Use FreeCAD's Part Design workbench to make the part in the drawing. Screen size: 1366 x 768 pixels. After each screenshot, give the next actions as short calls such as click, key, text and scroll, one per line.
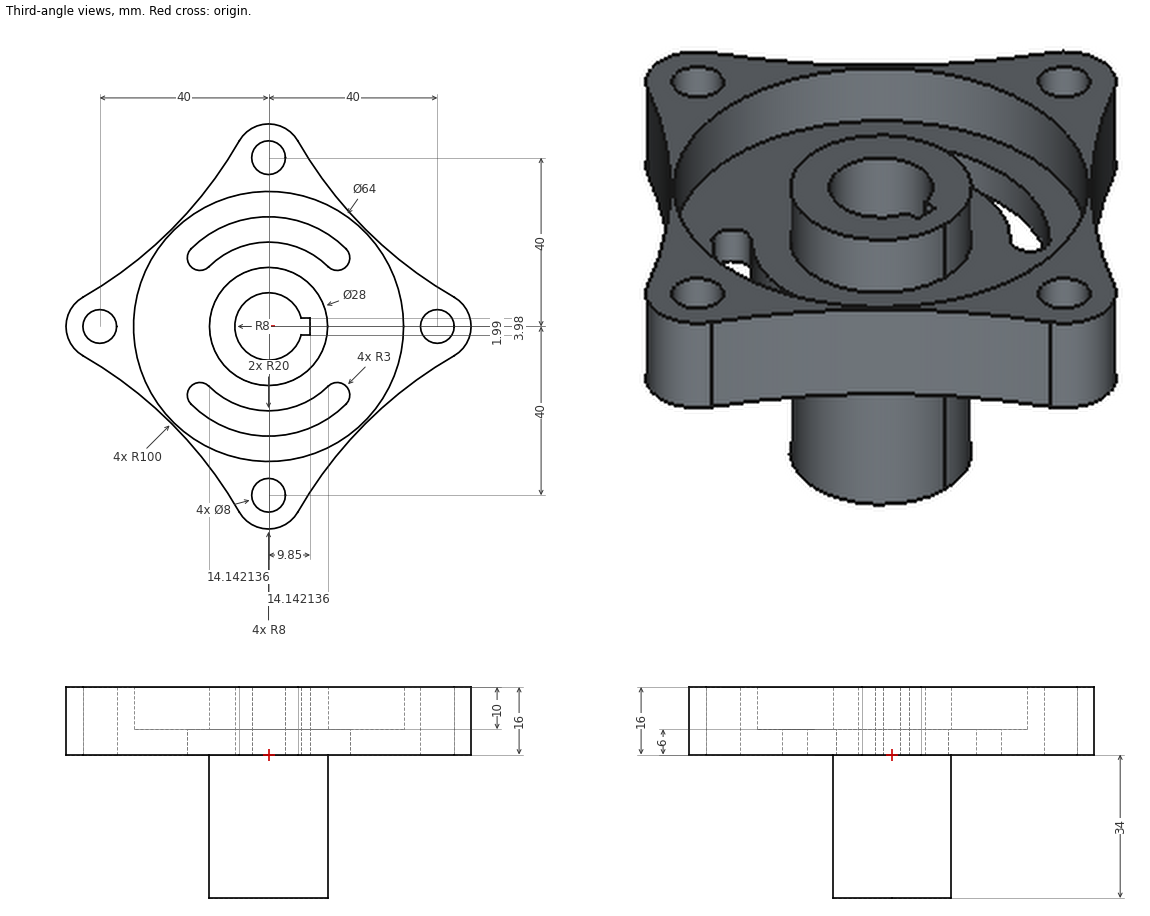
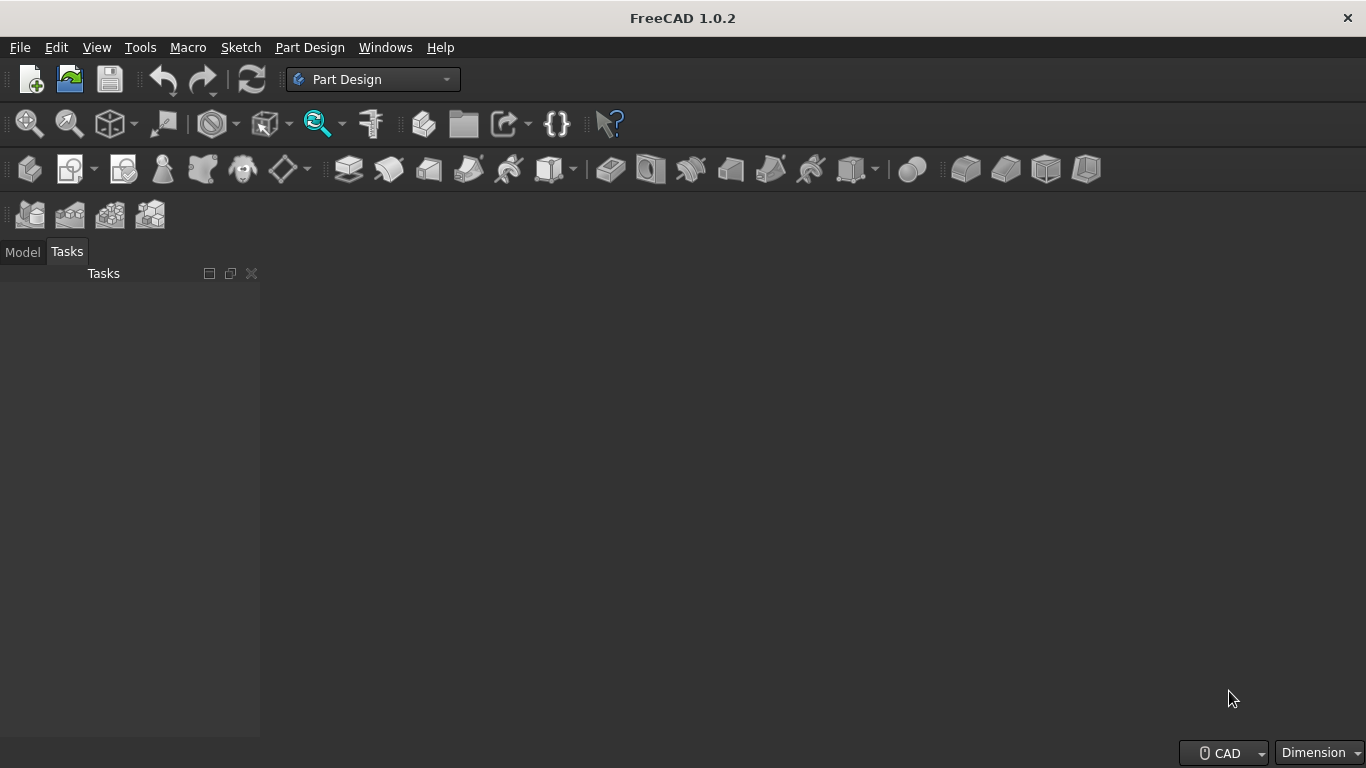
click(30, 80)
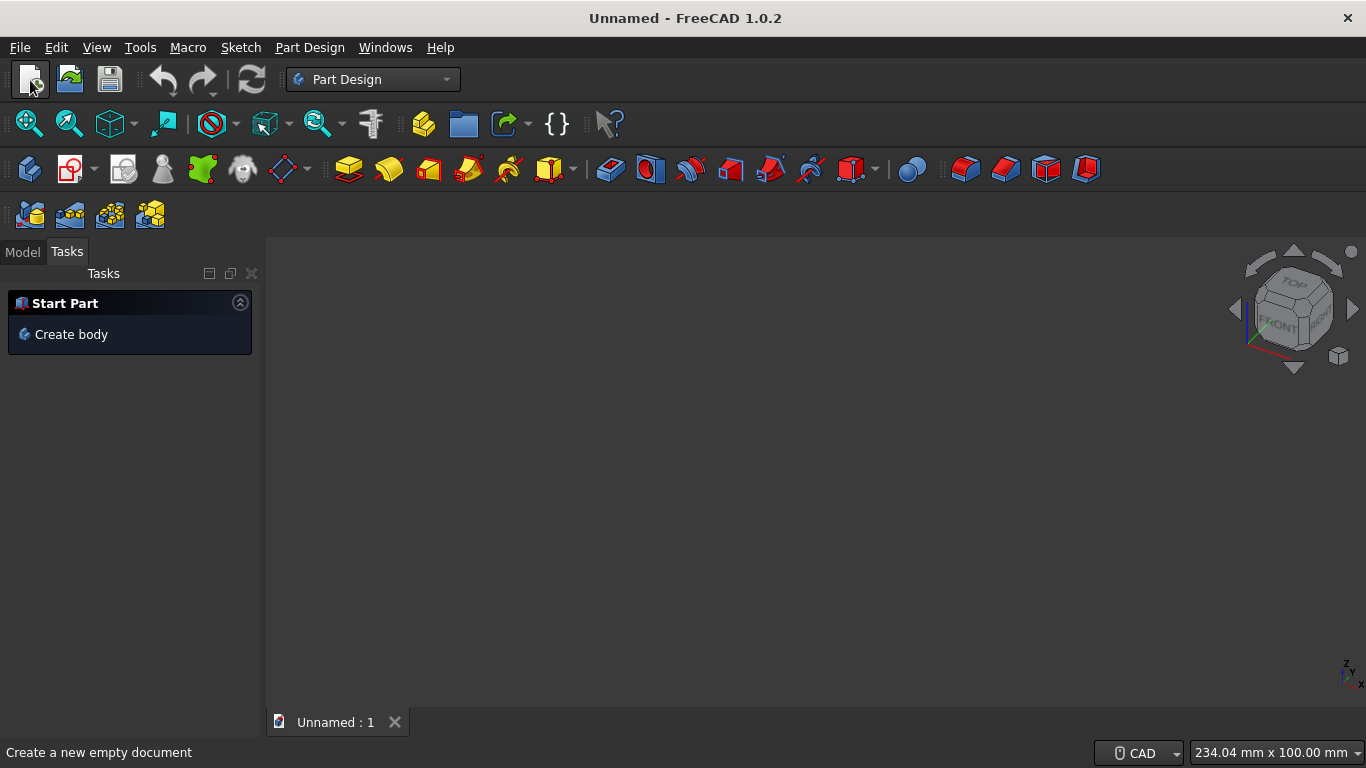
click(70, 170)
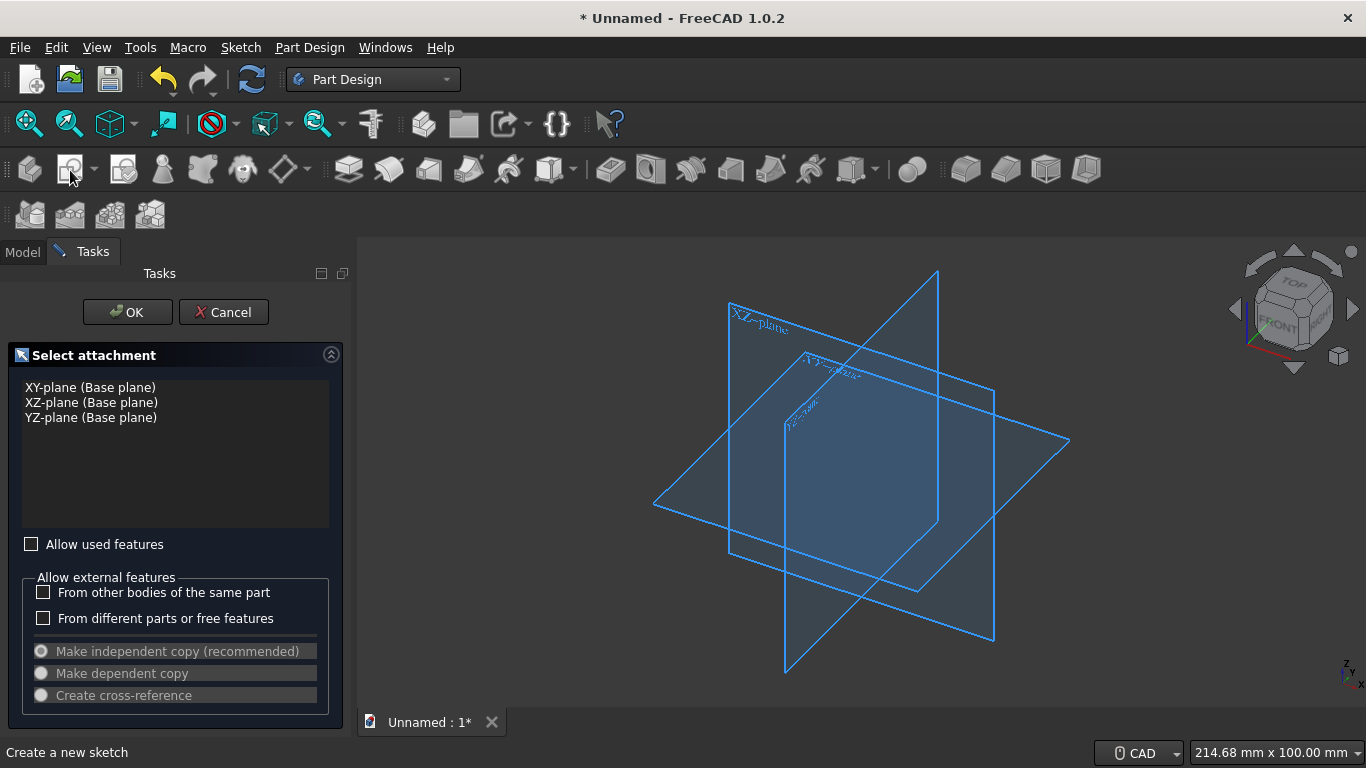
click(82, 388)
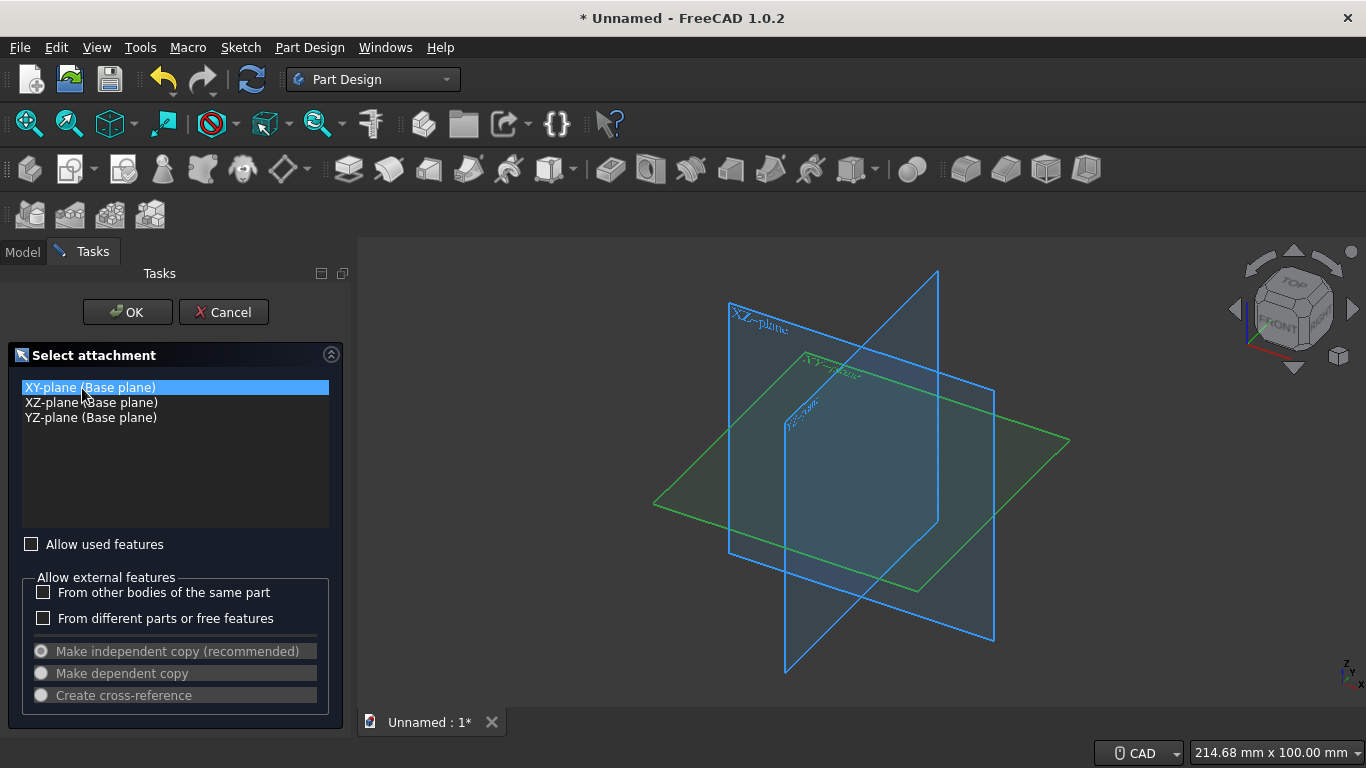
click(128, 312)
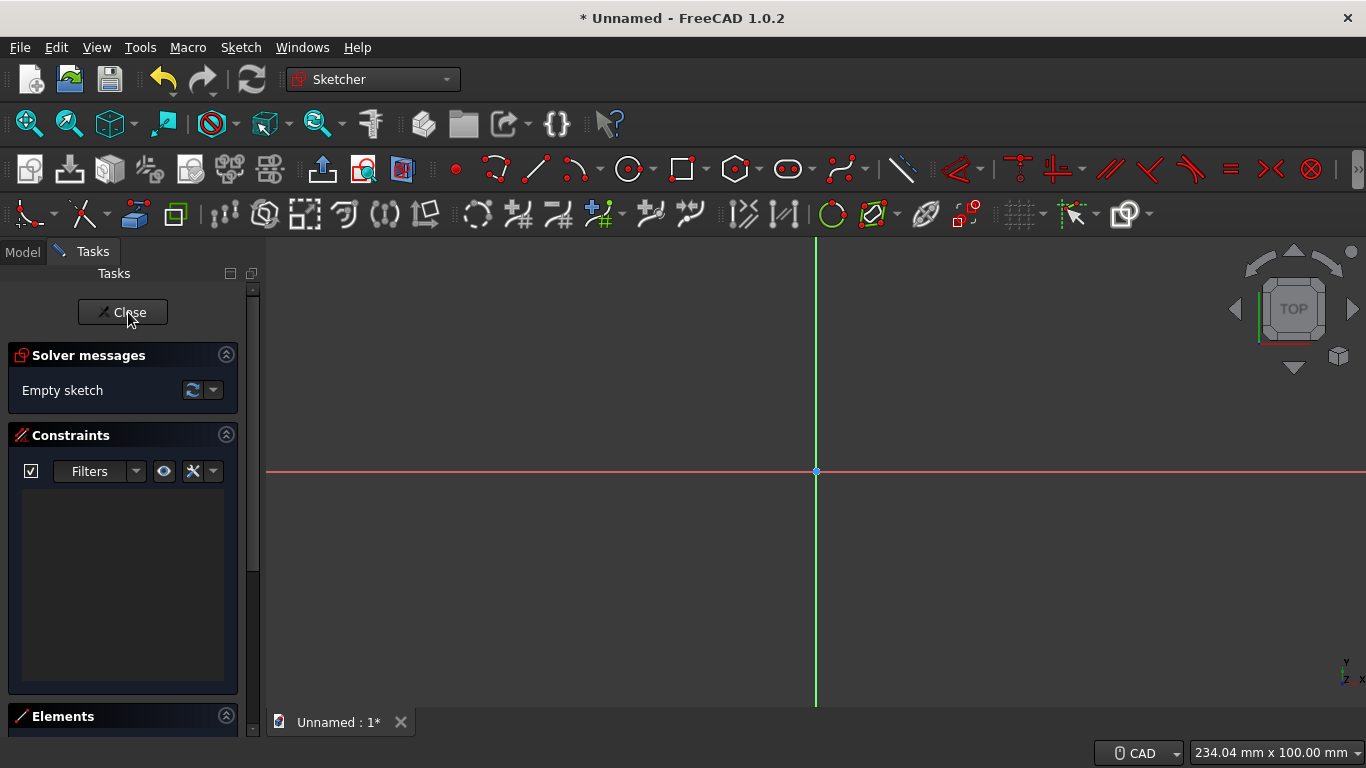
scroll(608, 472, down, 2)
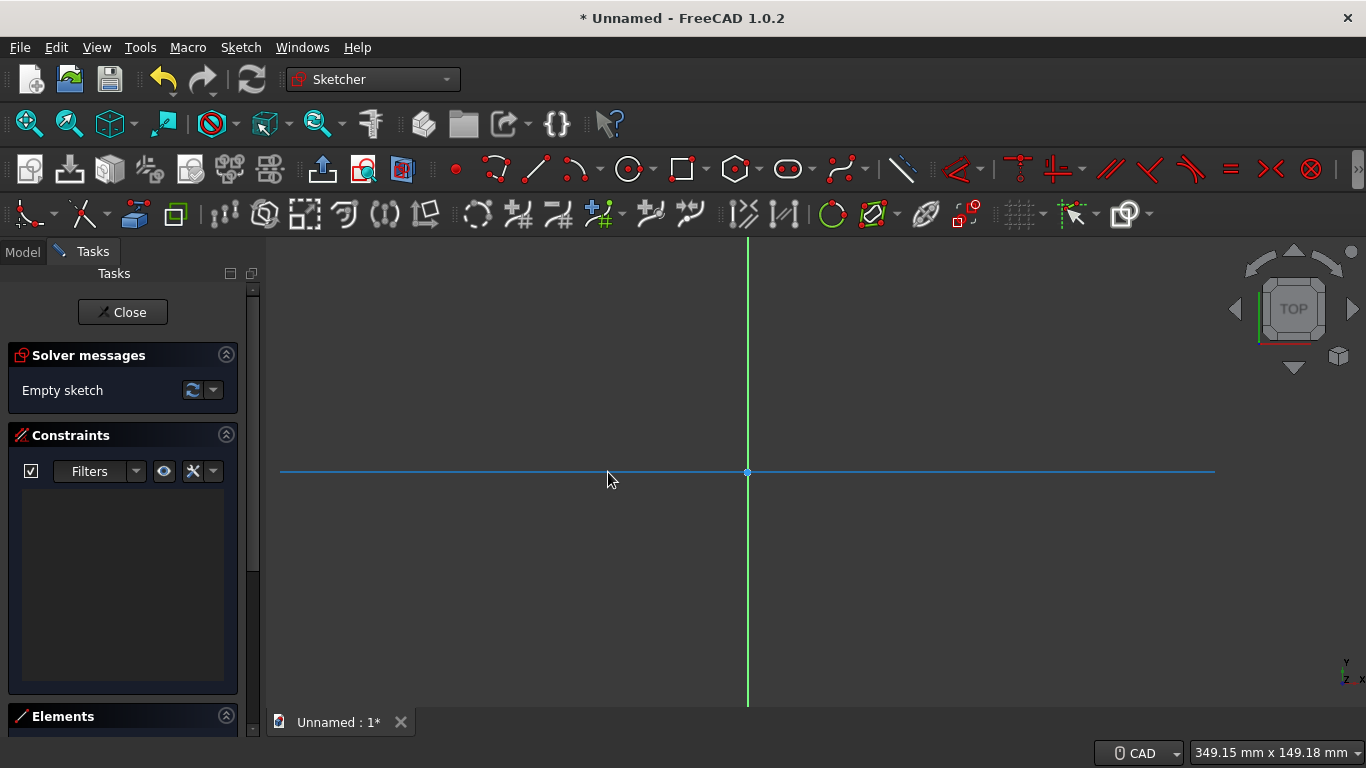
click(602, 170)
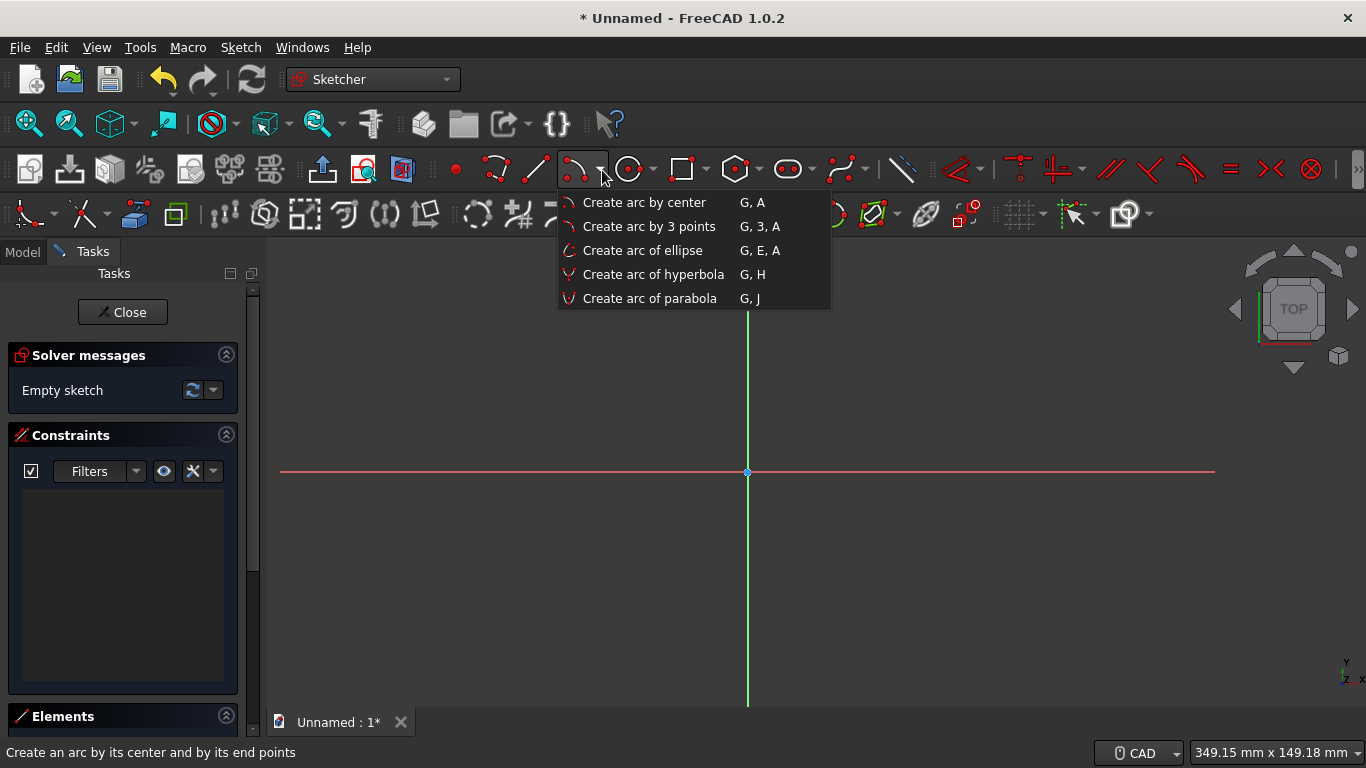
click(694, 226)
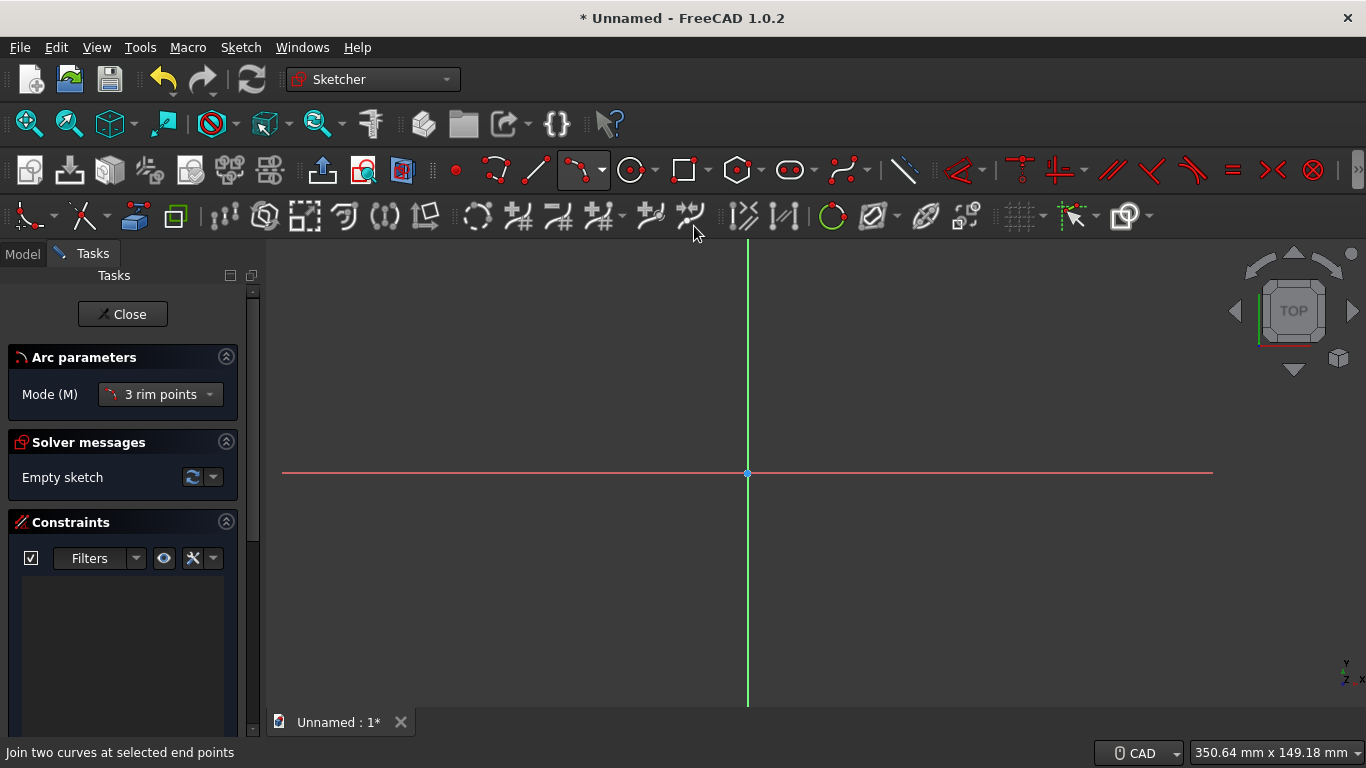
click(610, 495)
click(726, 611)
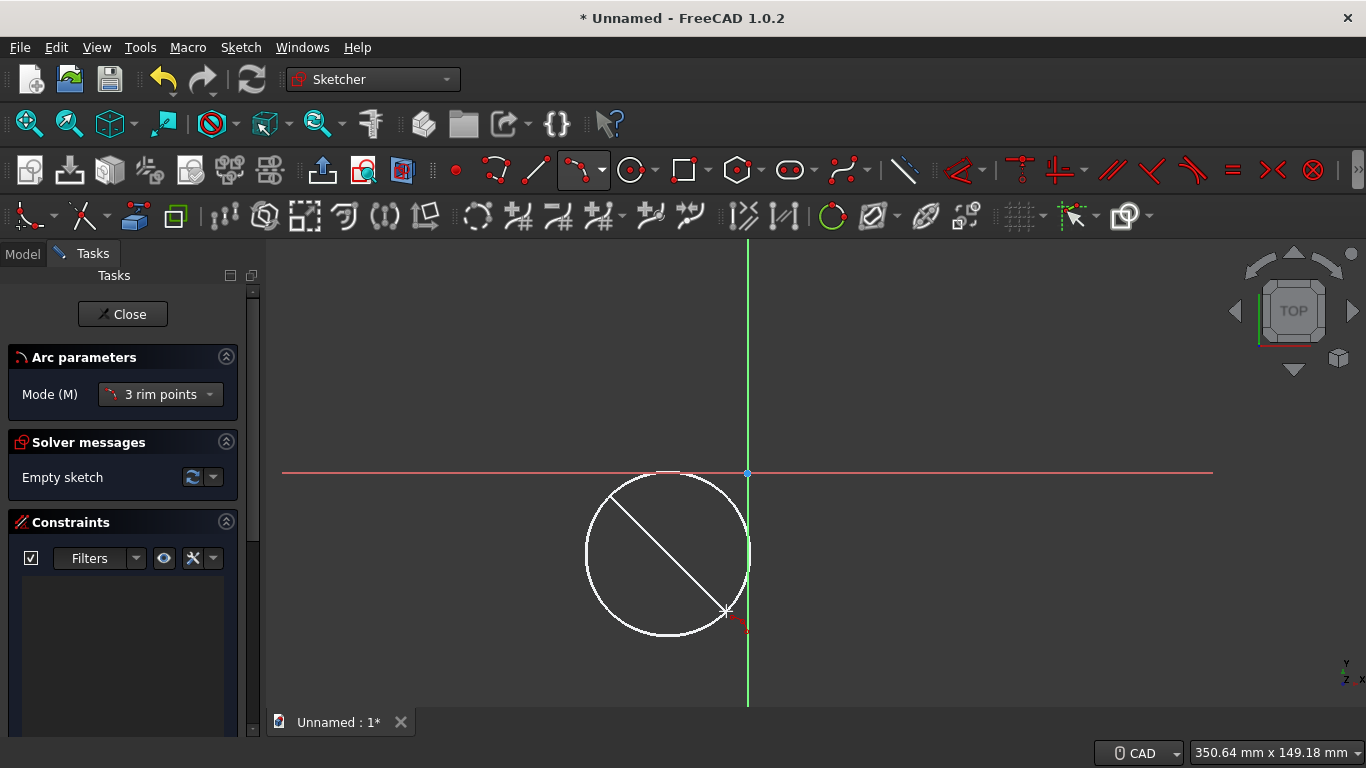
scroll(676, 545, up, 2)